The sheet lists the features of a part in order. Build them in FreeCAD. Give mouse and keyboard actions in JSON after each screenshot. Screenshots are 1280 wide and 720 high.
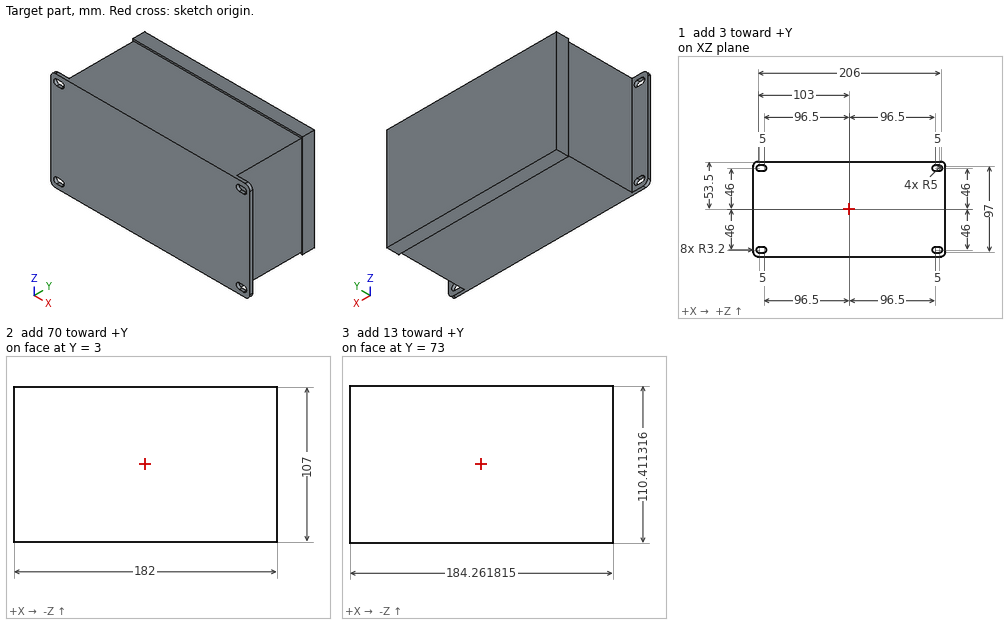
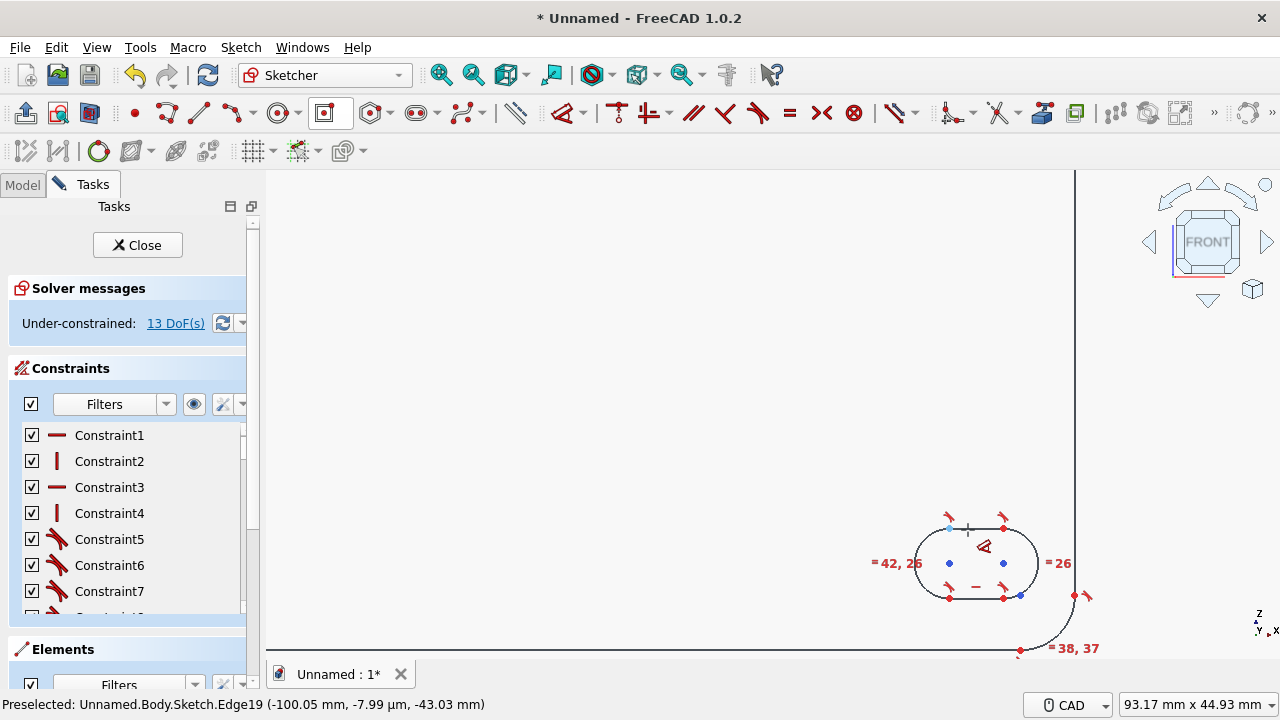
{"action": "left_click", "coordinate": [966, 529]}
{"action": "left_click", "coordinate": [976, 563]}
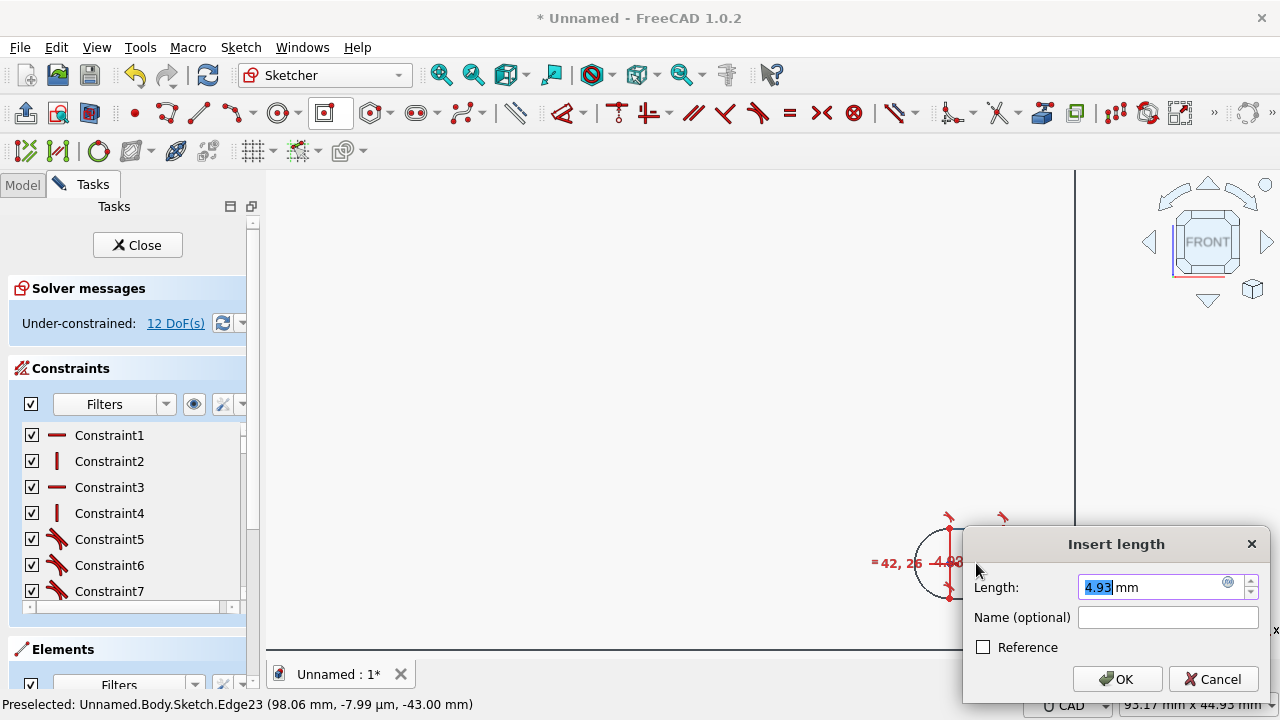
{"action": "type", "text": "5"}
{"action": "key", "text": "Return"}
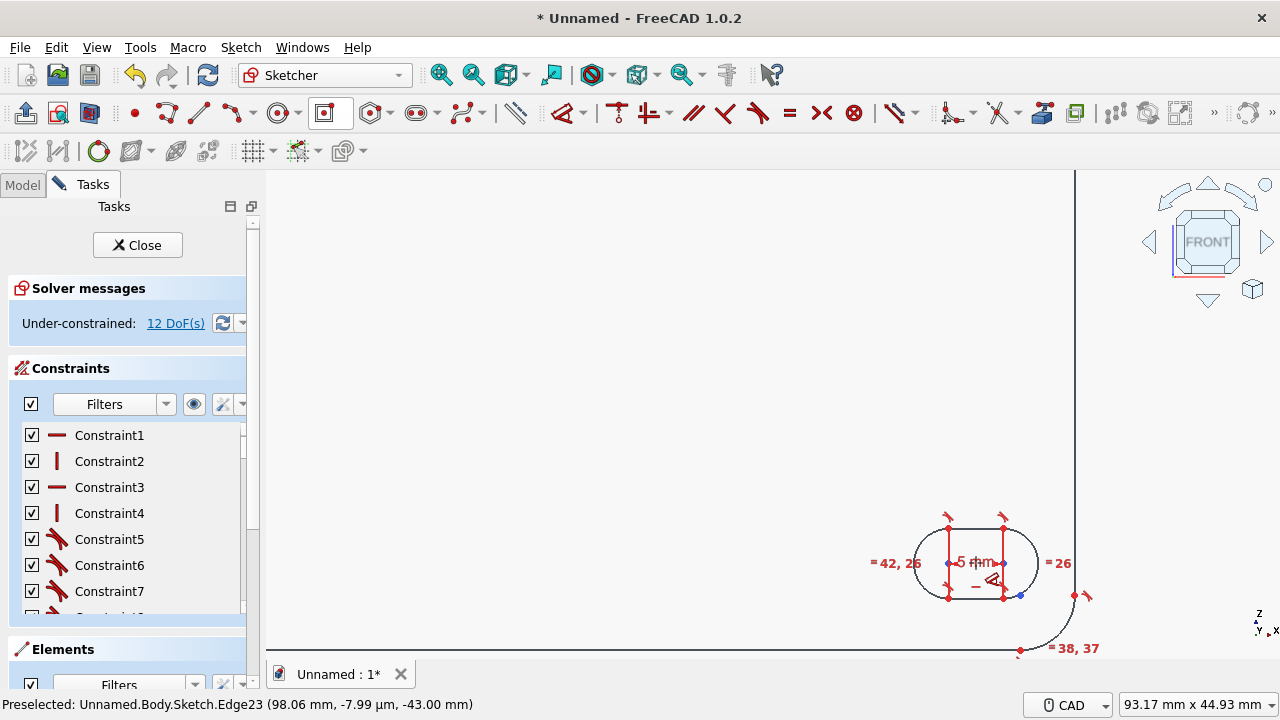
{"action": "scroll", "coordinate": [968, 530], "scroll_direction": "down", "scroll_amount": 7}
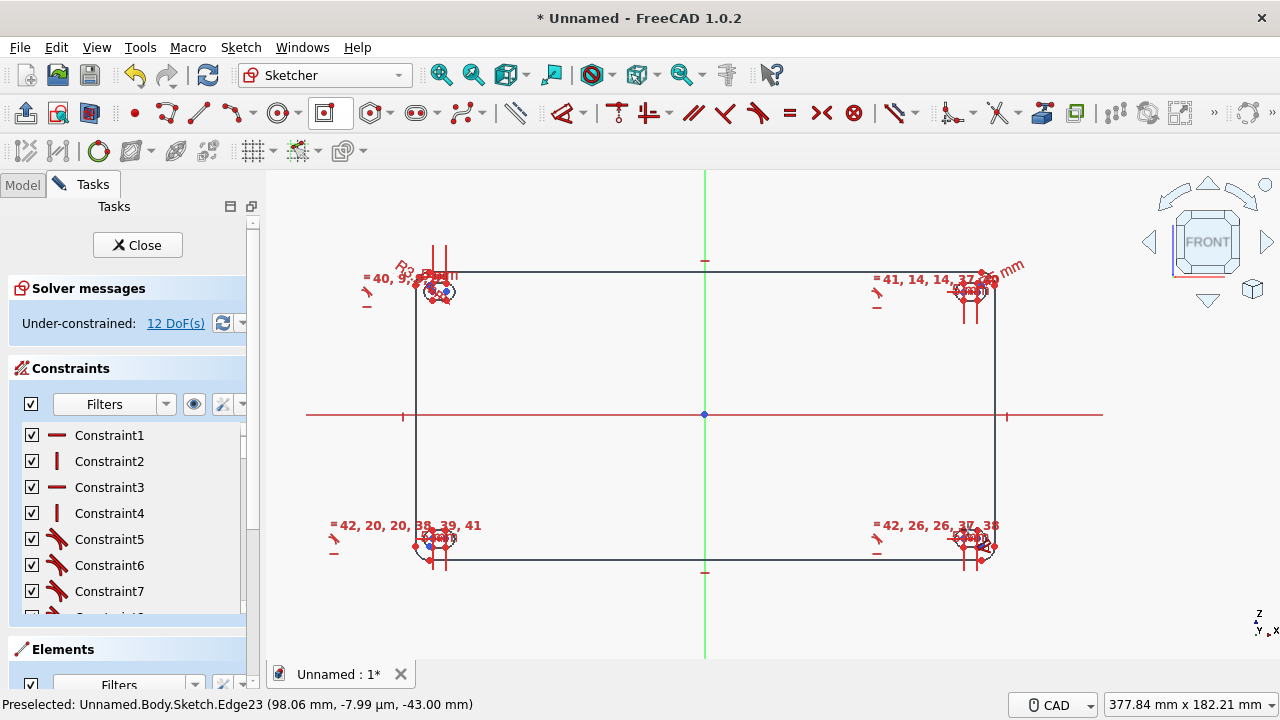
{"action": "left_click", "coordinate": [995, 468]}
{"action": "left_click", "coordinate": [1029, 356]}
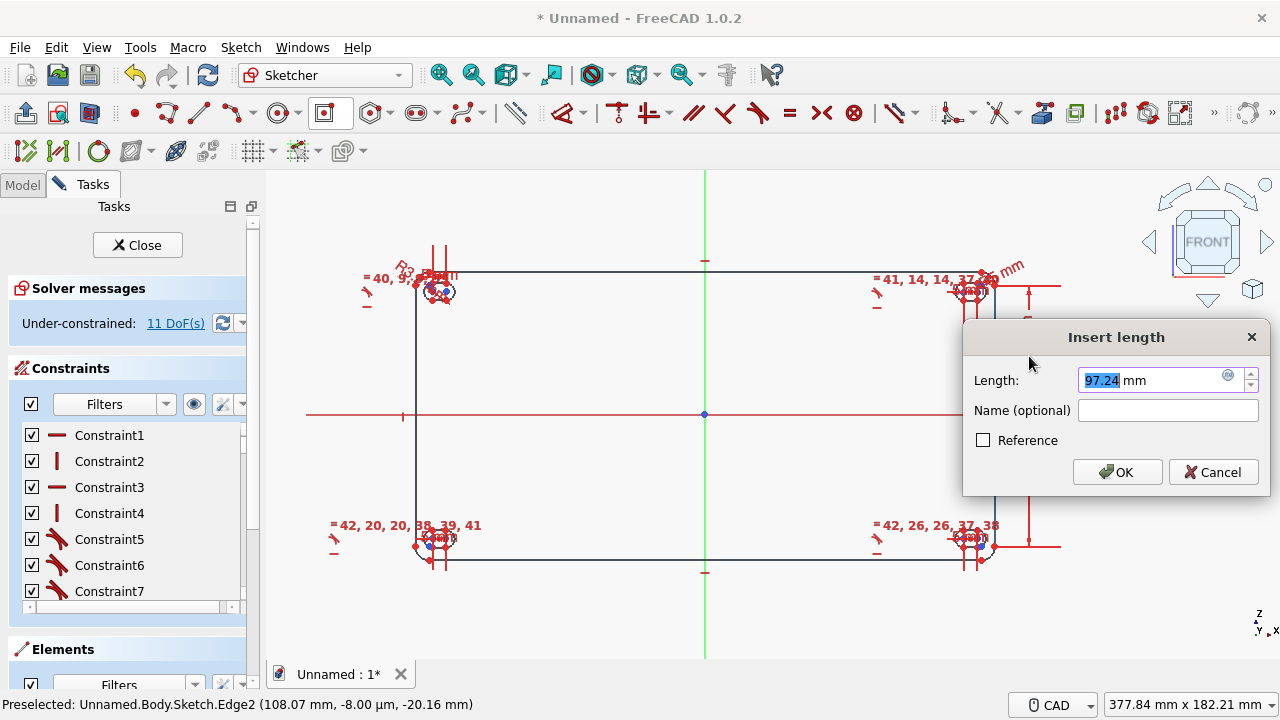
{"action": "type", "text": "97"}
{"action": "key", "text": "Return"}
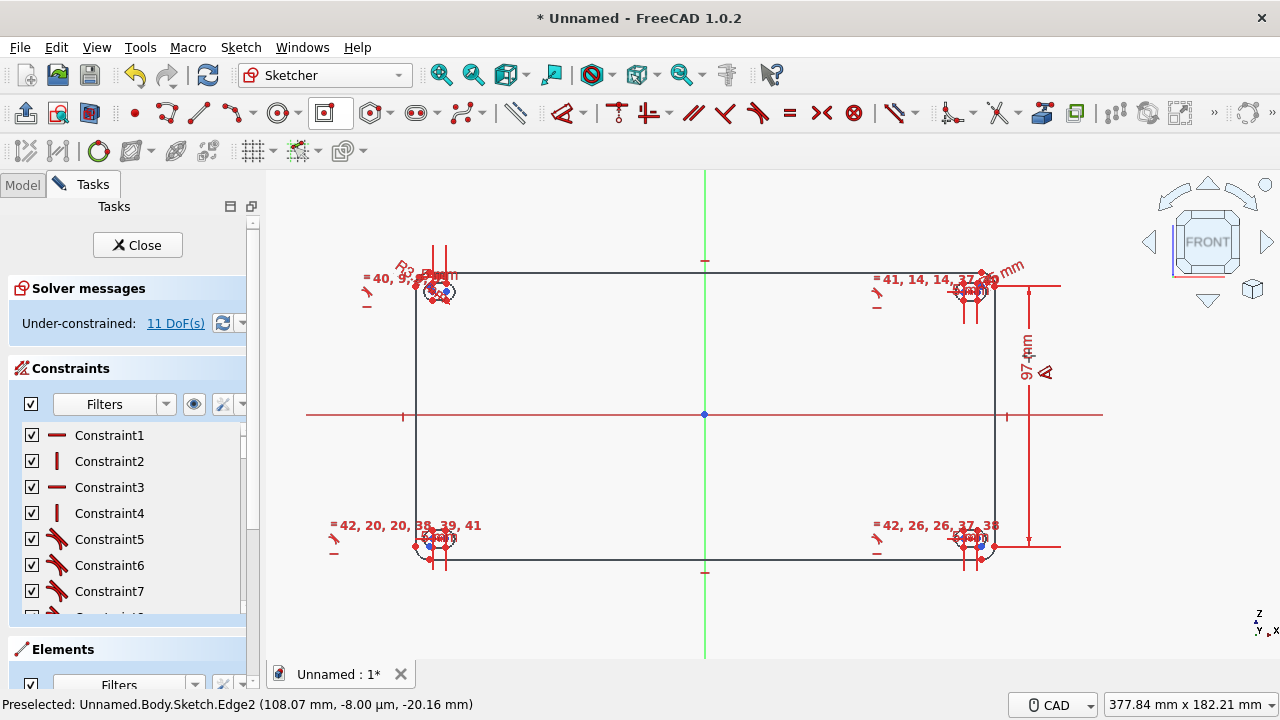
{"action": "left_click", "coordinate": [595, 273]}
{"action": "left_click", "coordinate": [578, 239]}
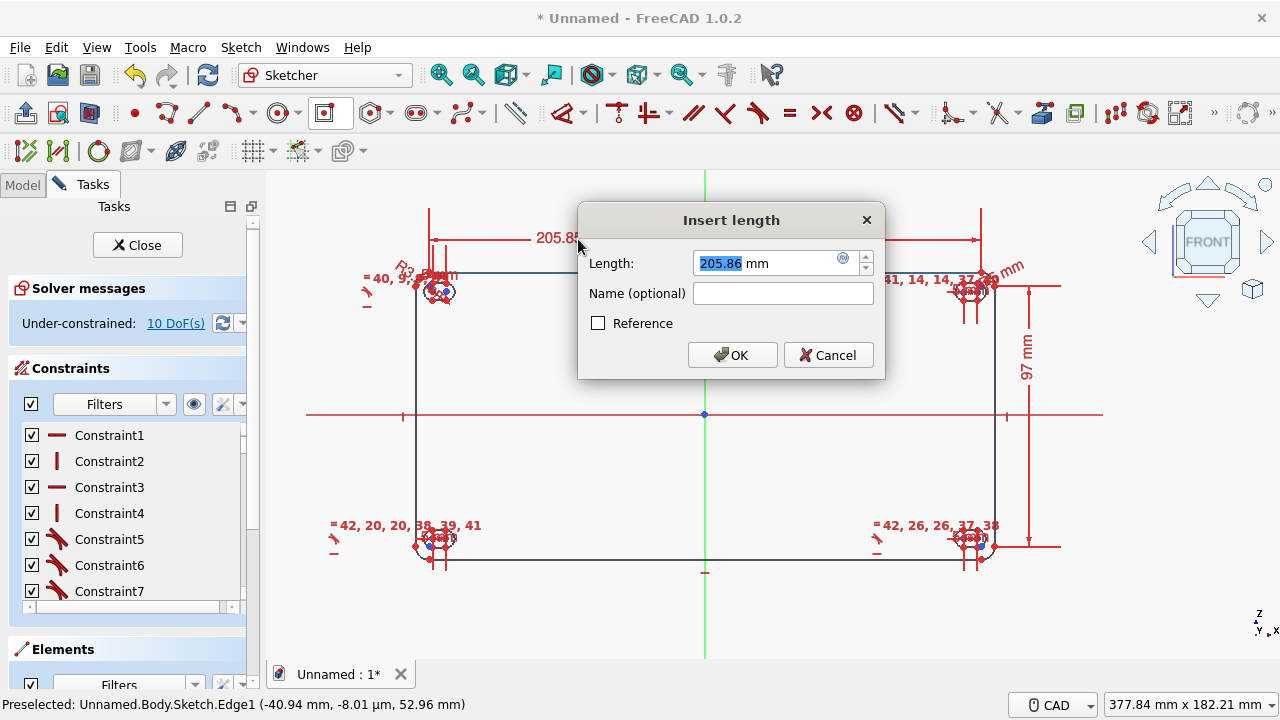
{"action": "type", "text": "206"}
{"action": "key", "text": "Return"}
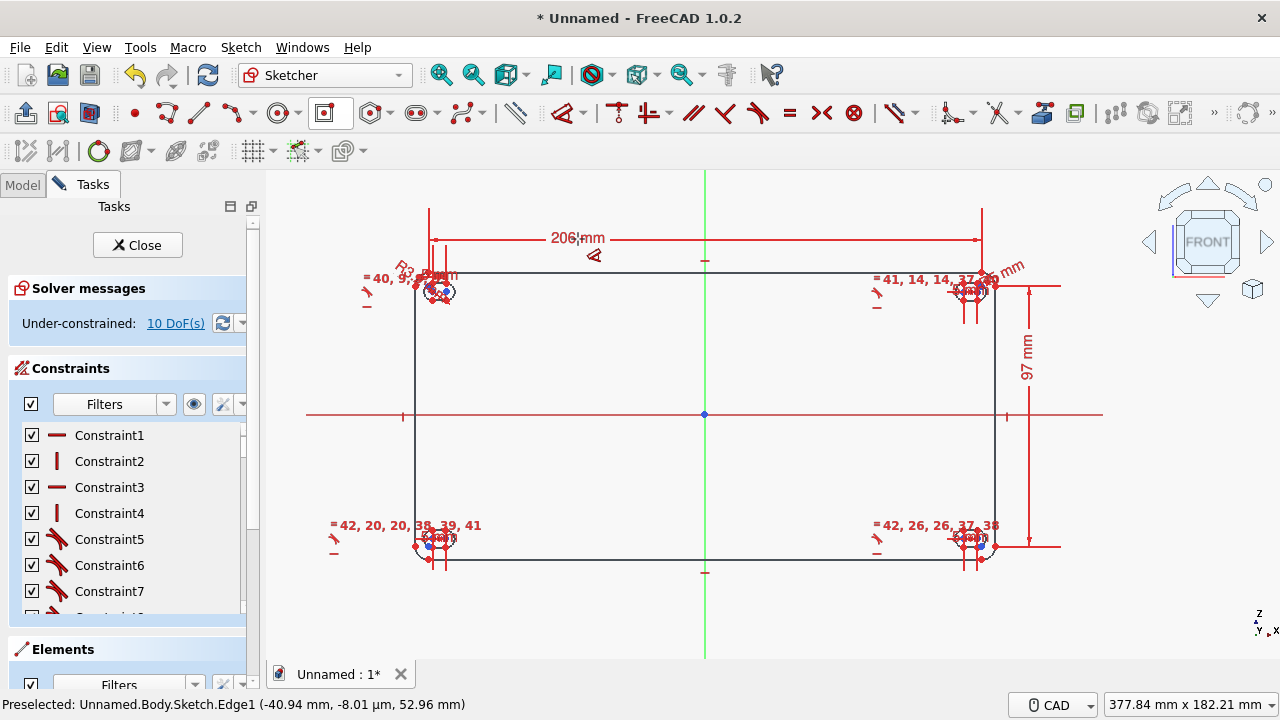
{"action": "scroll", "coordinate": [433, 292], "scroll_direction": "up", "scroll_amount": 3}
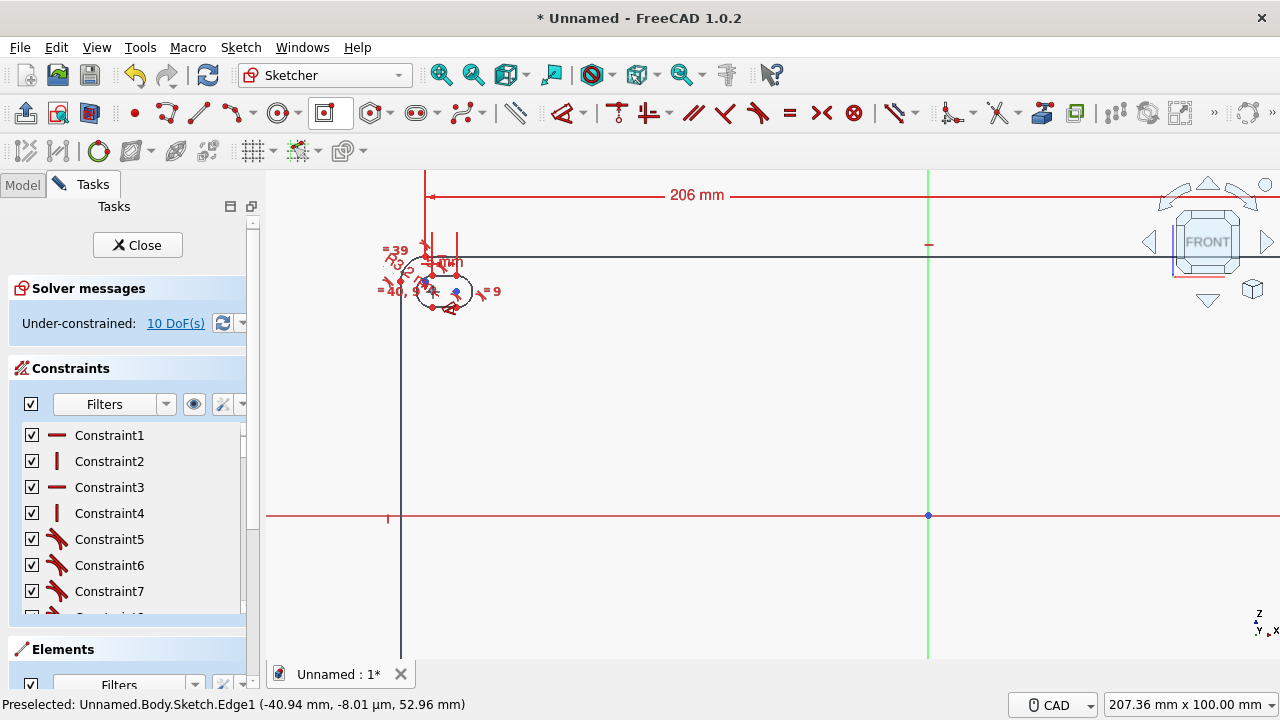
{"action": "left_click", "coordinate": [432, 292]}
{"action": "left_click", "coordinate": [962, 404]}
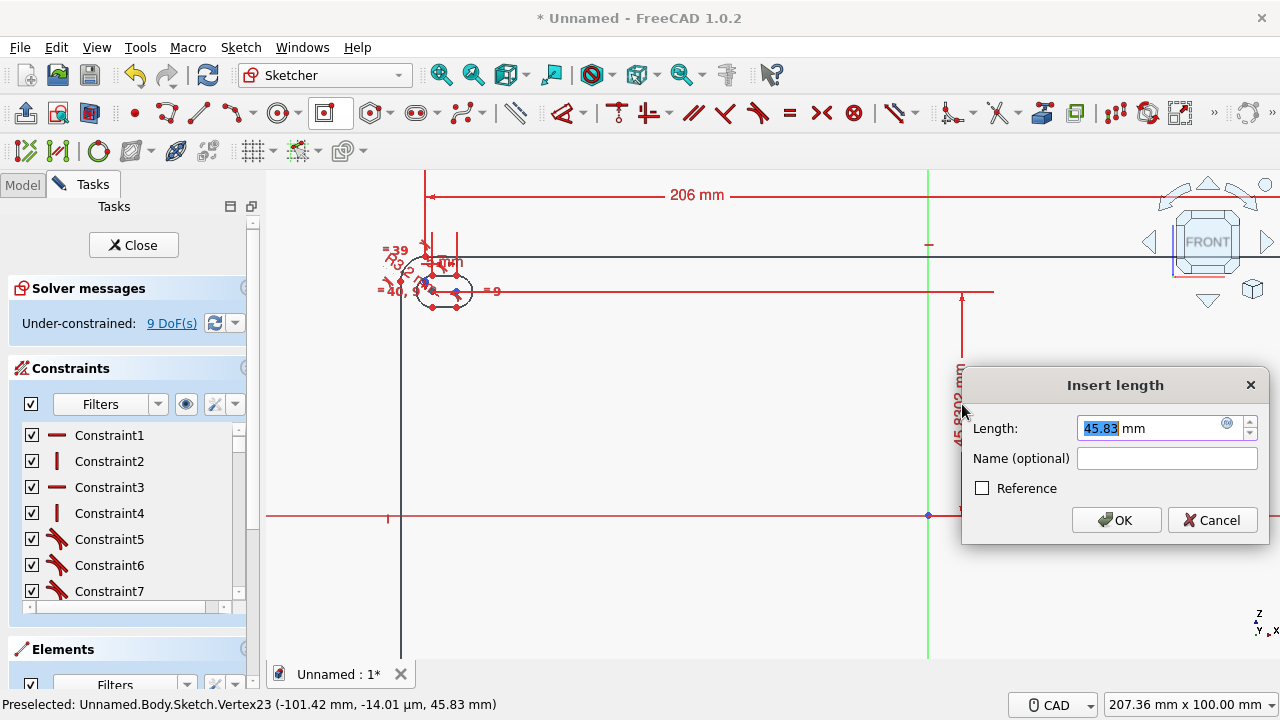
{"action": "type", "text": "46"}
{"action": "key", "text": "Return"}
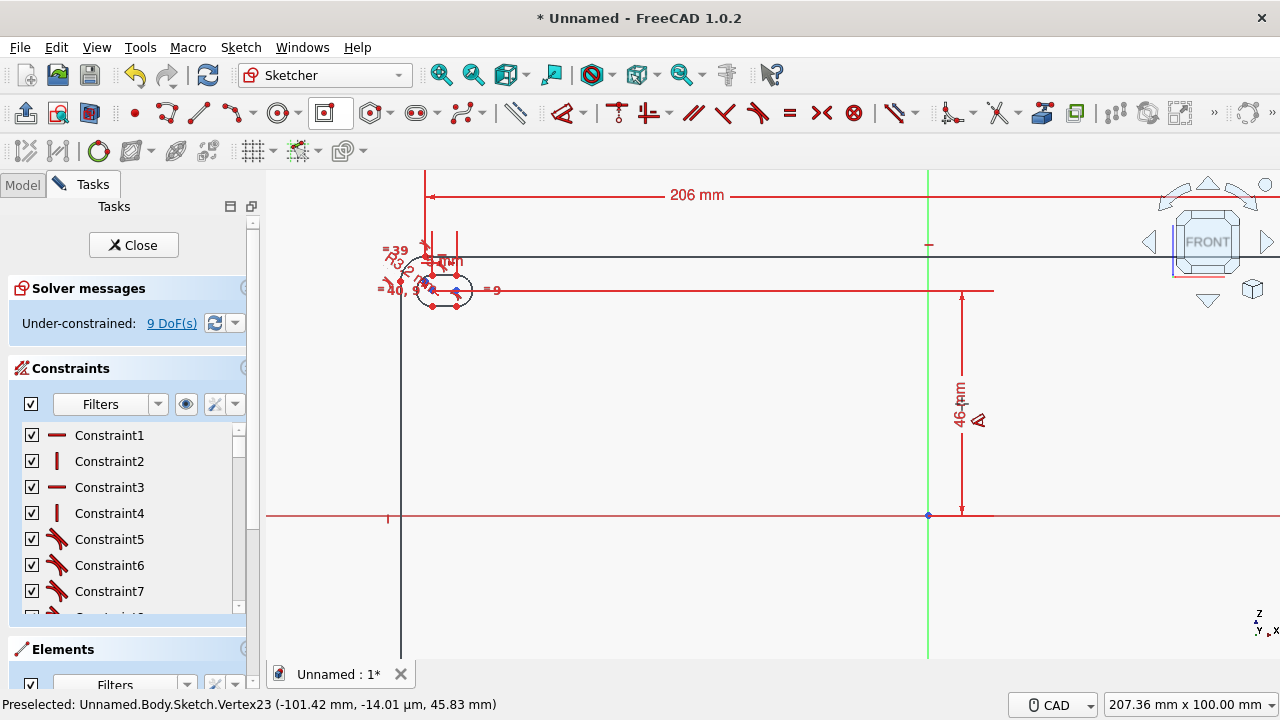
{"action": "scroll", "coordinate": [432, 291], "scroll_direction": "down", "scroll_amount": 3}